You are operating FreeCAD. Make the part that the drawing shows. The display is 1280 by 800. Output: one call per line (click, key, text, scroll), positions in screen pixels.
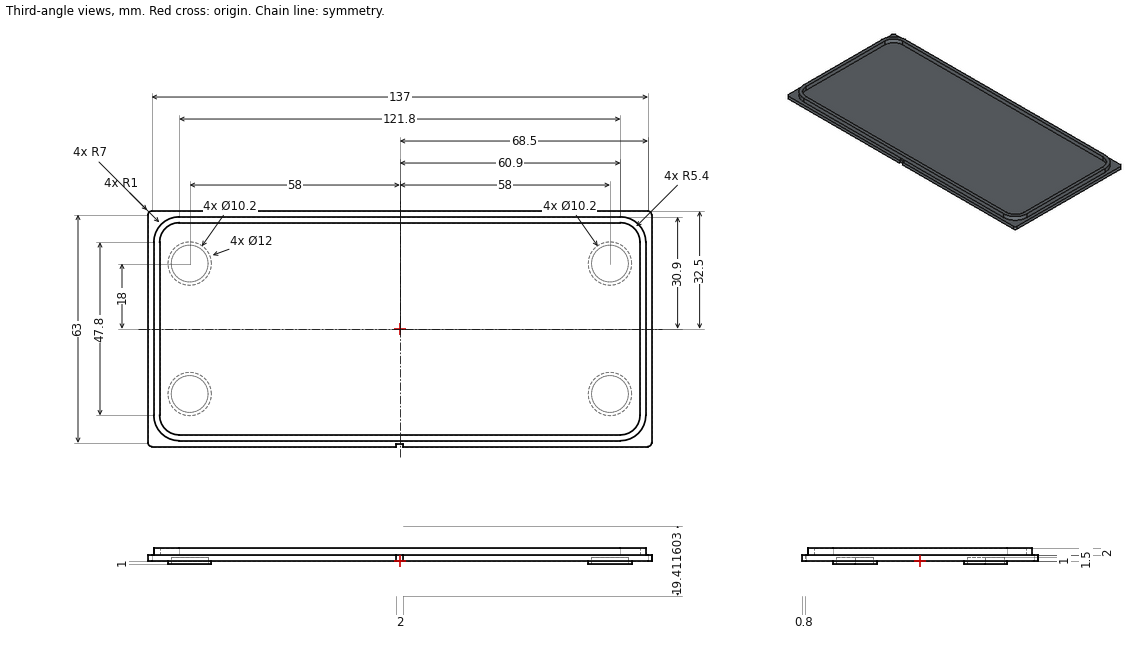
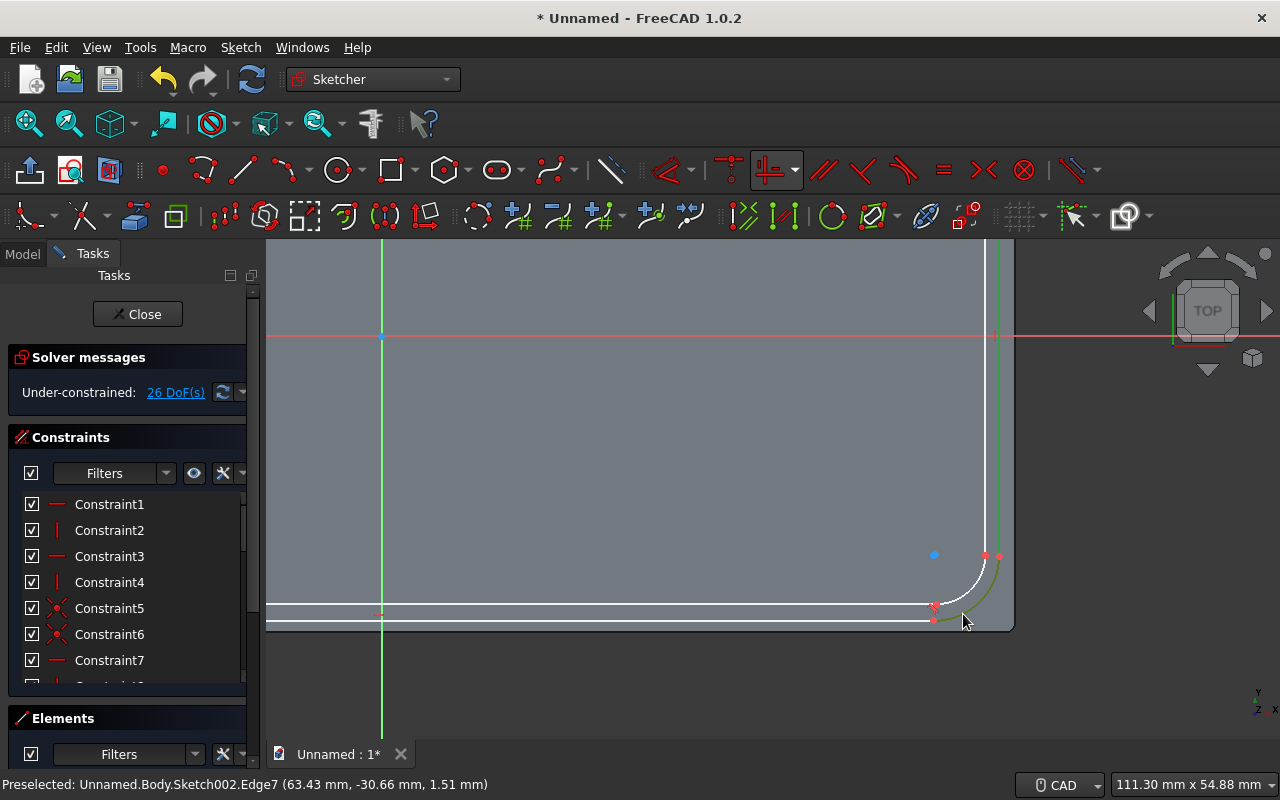
click(904, 170)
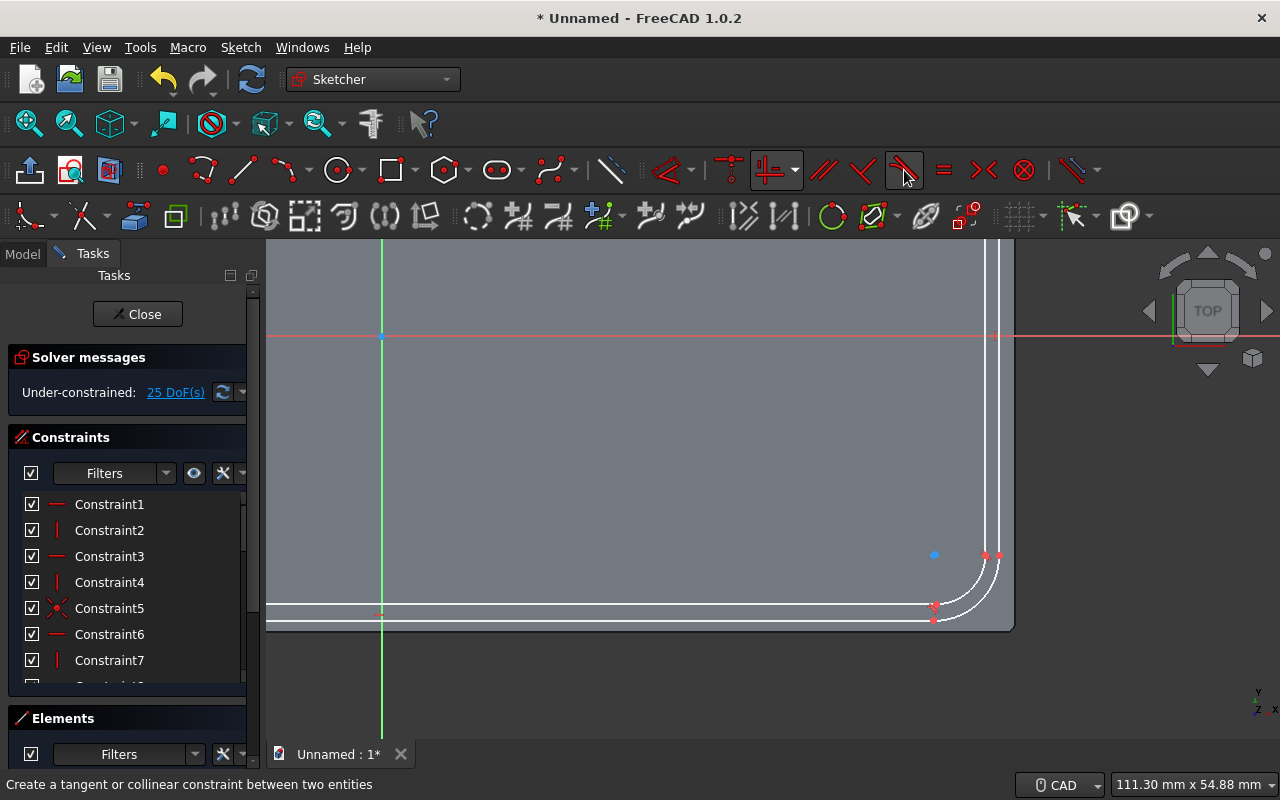
click(999, 425)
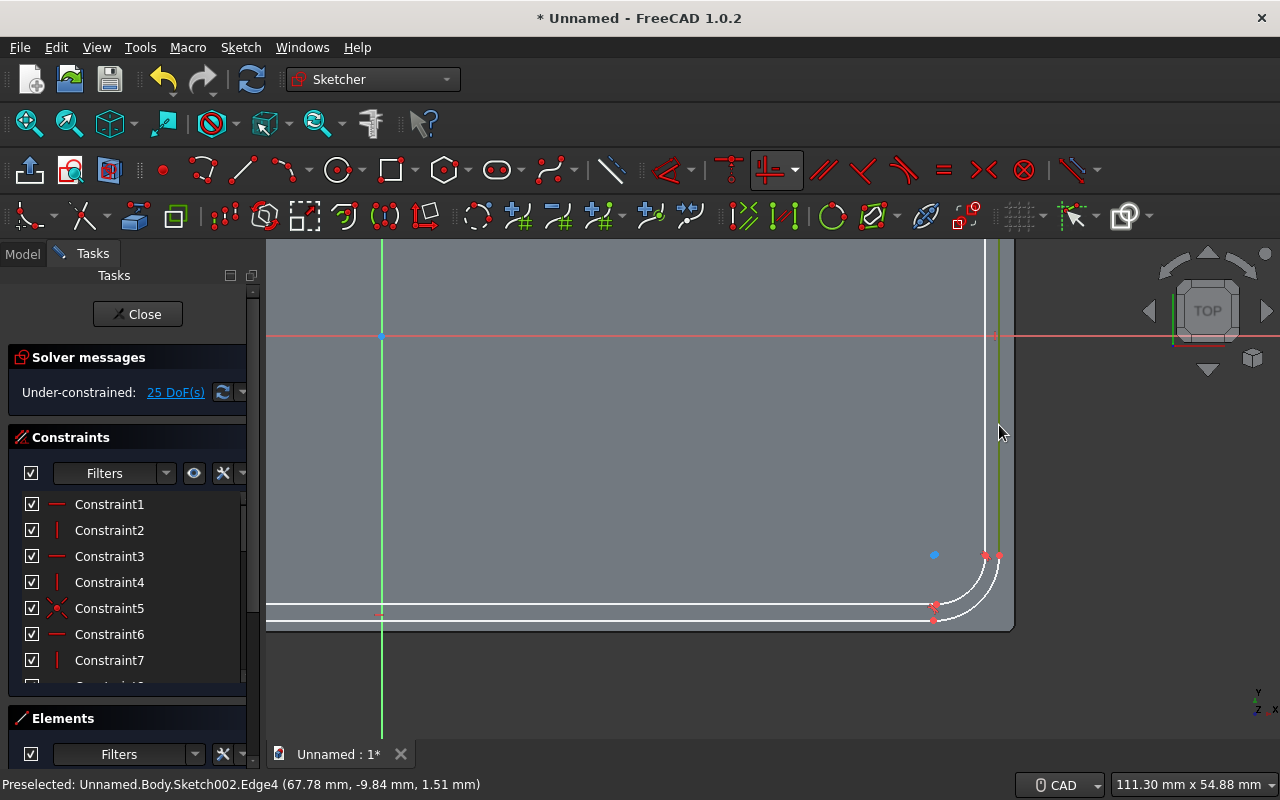
scroll(968, 614, down, 4)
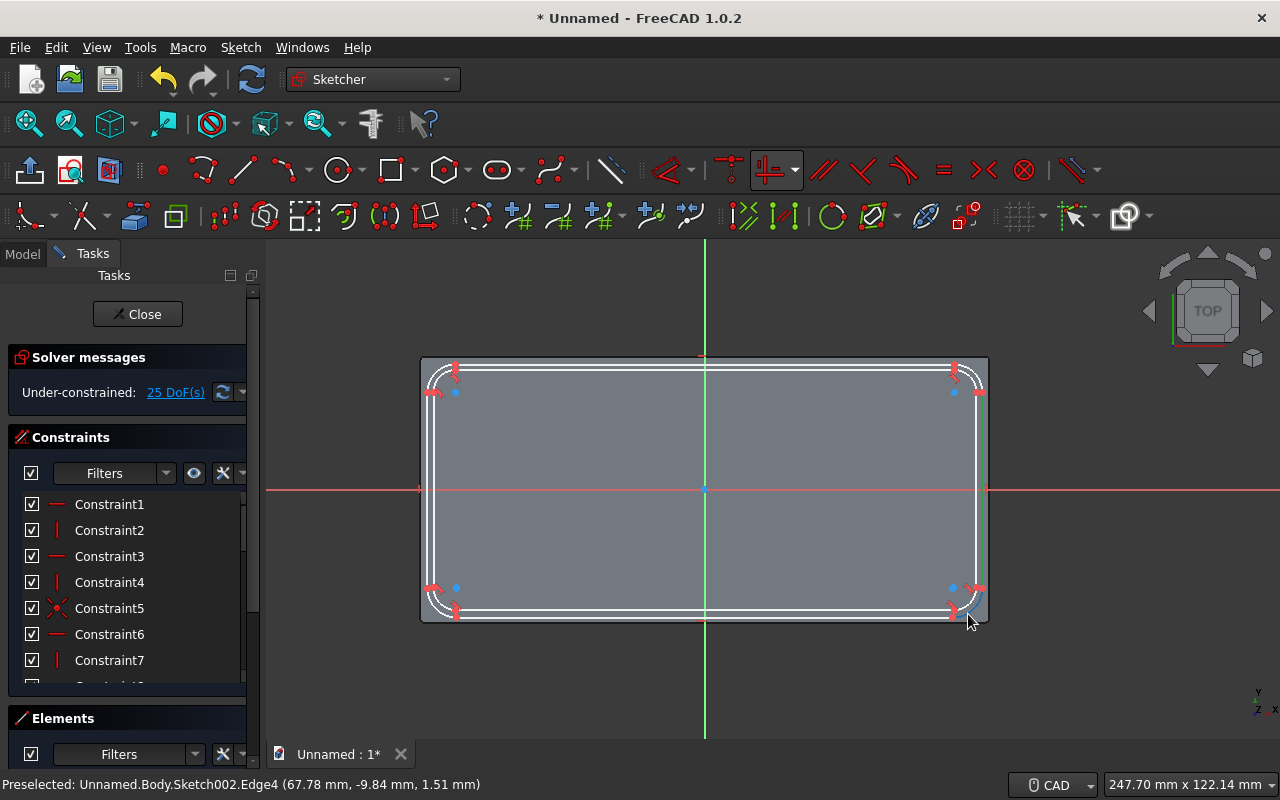
scroll(979, 380, up, 5)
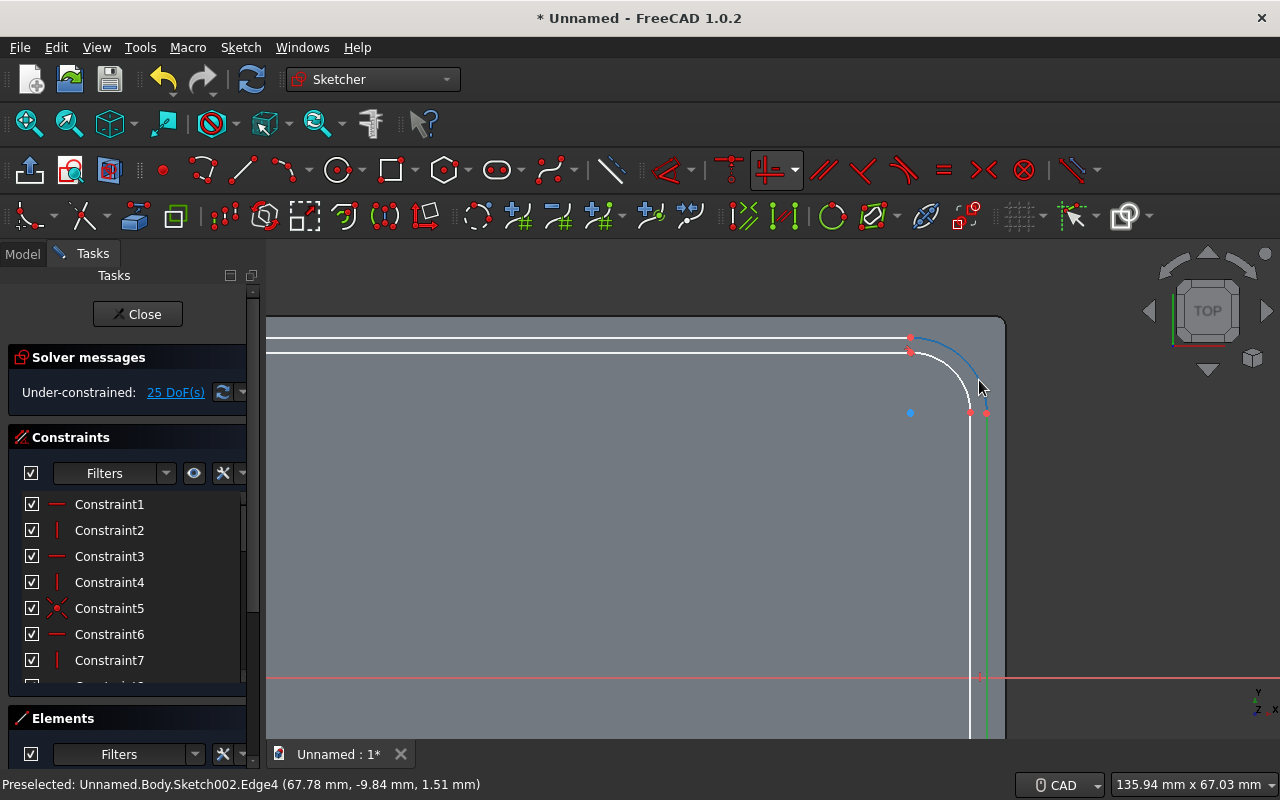
click(979, 379)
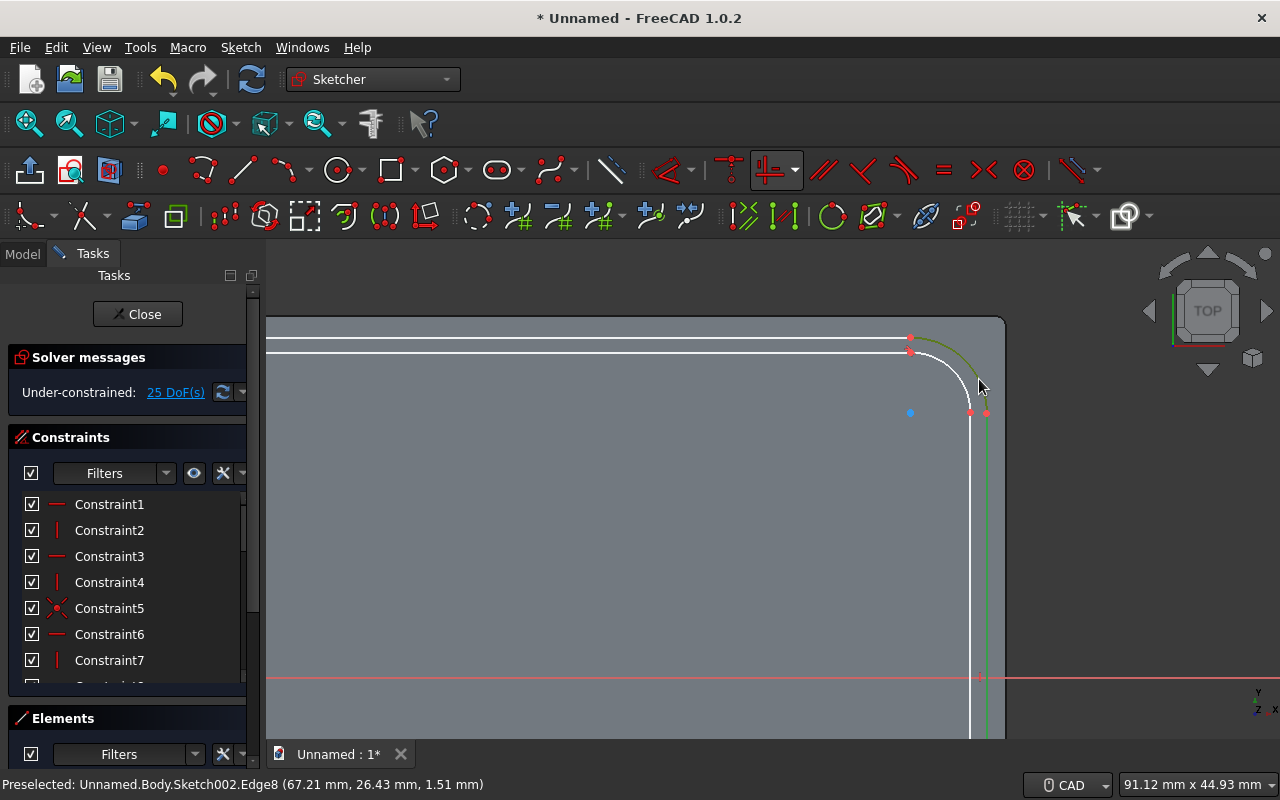
click(904, 170)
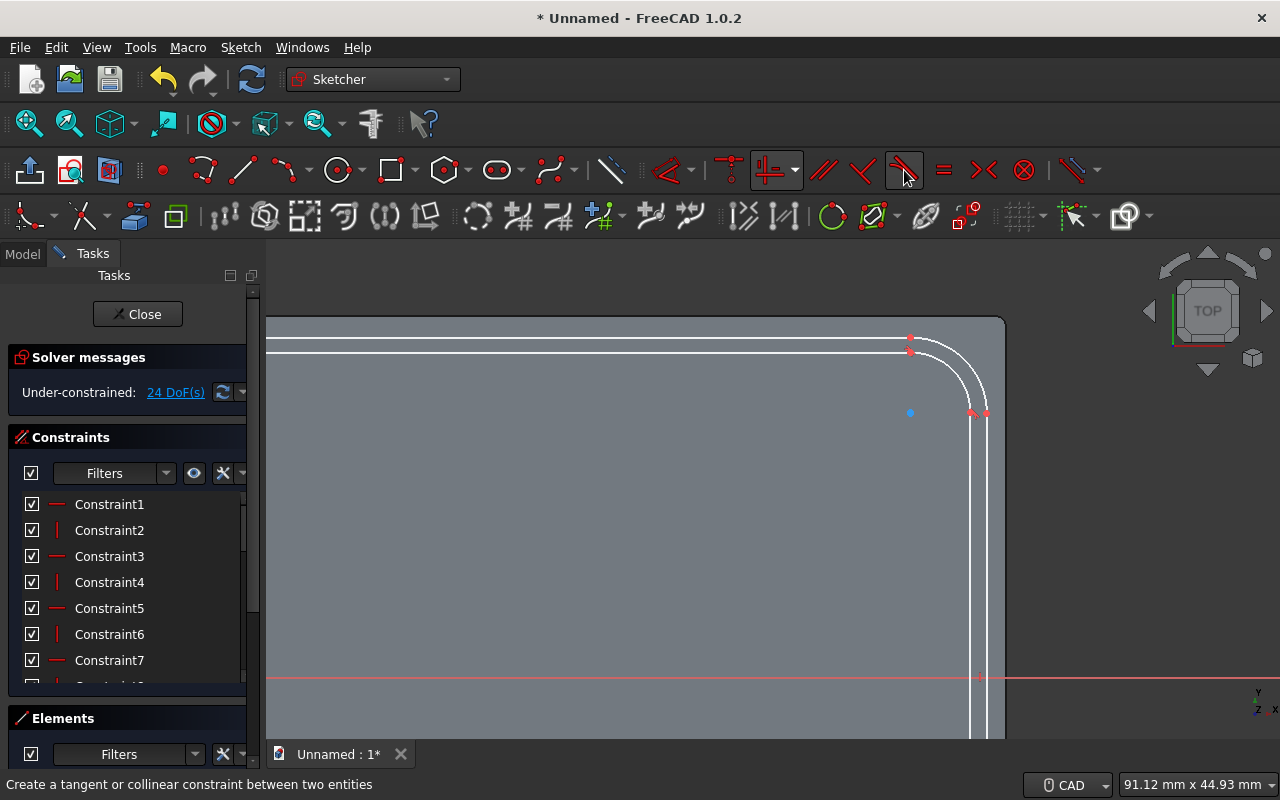
click(504, 353)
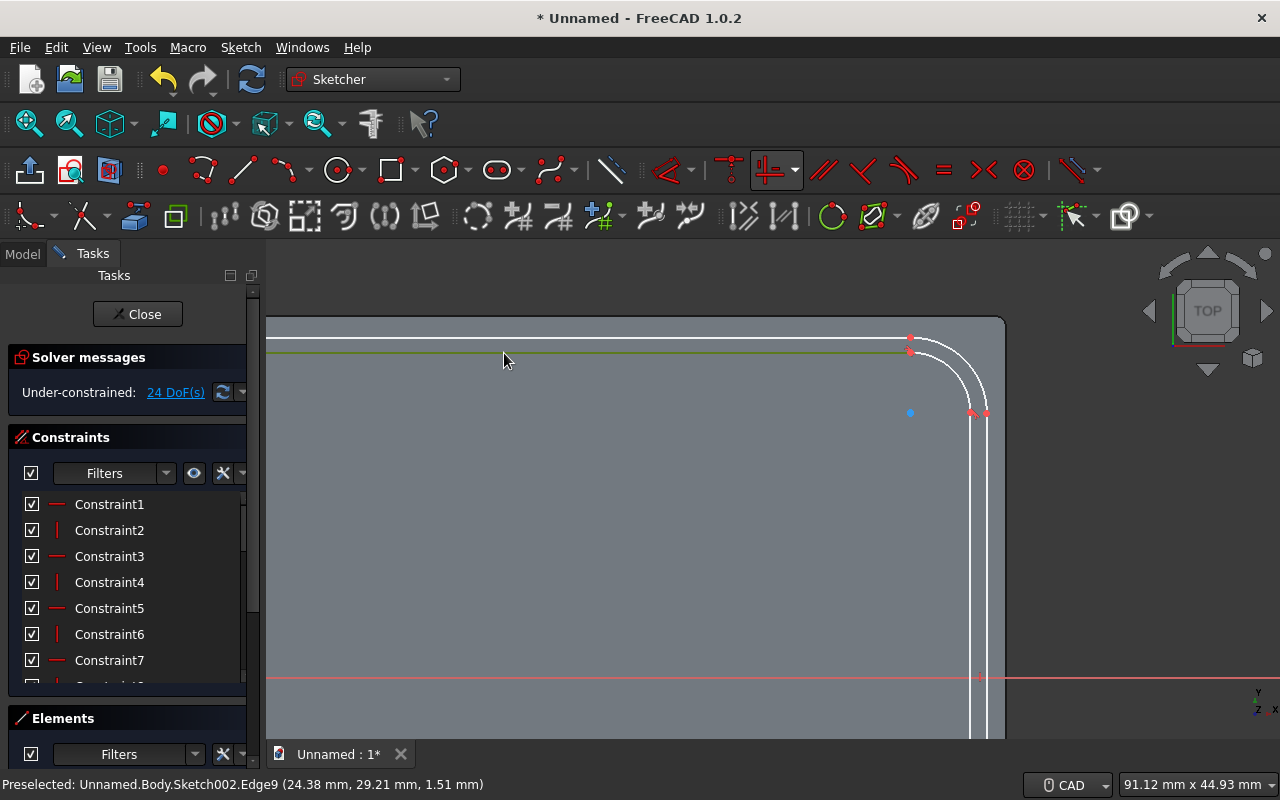
click(964, 385)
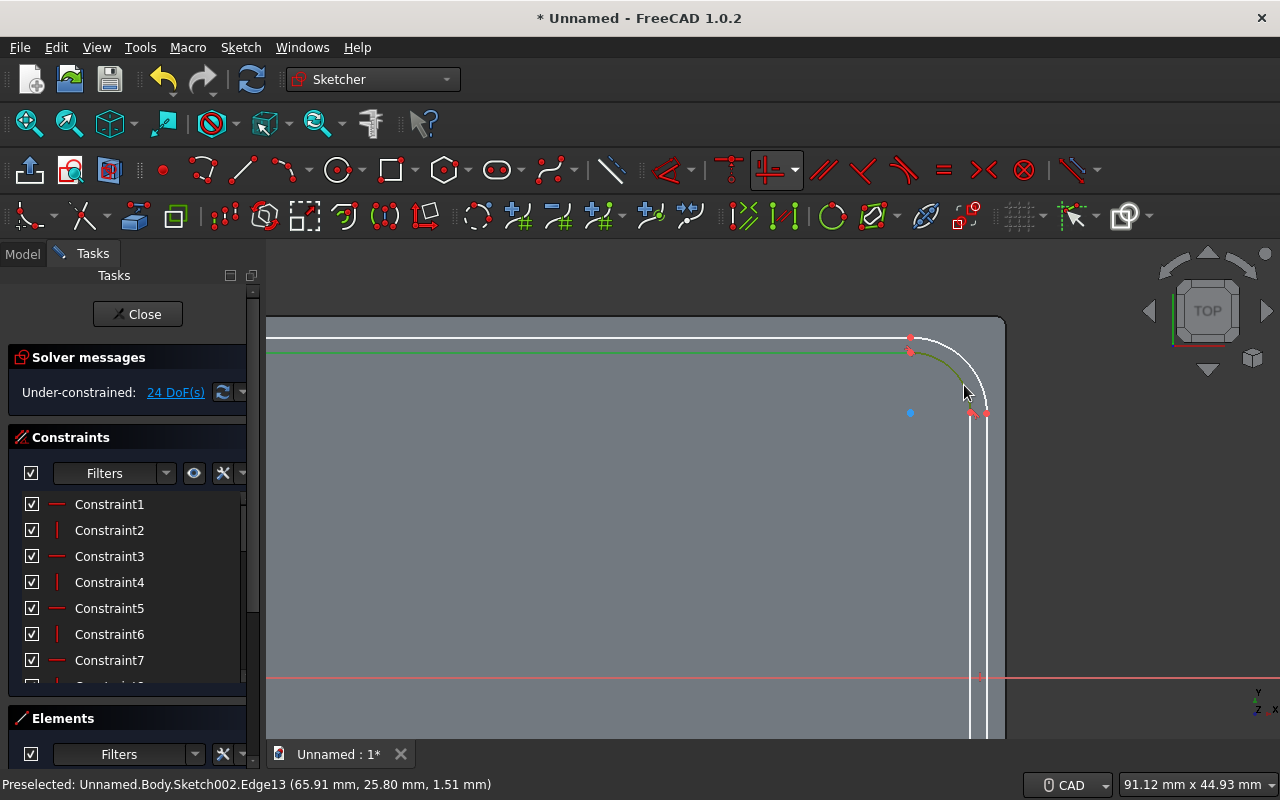
click(904, 170)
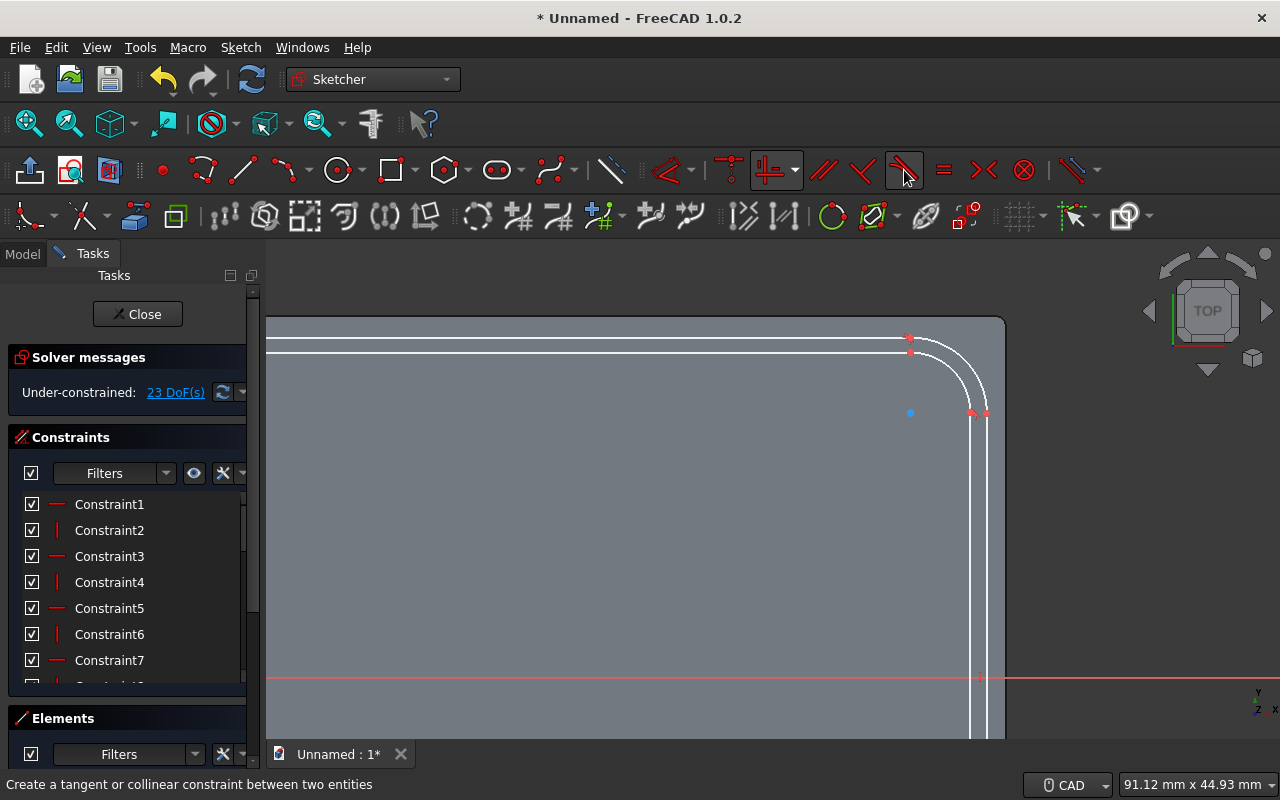
click(504, 353)